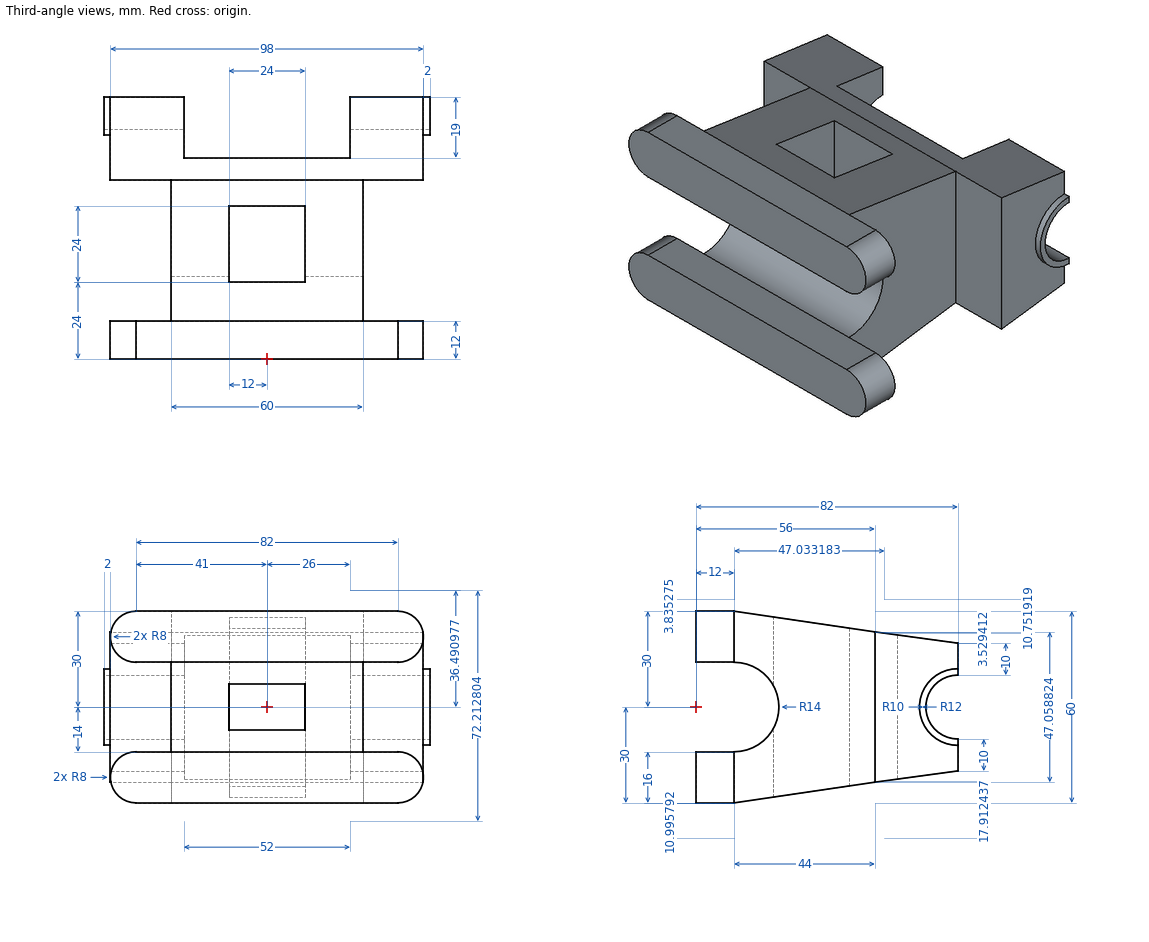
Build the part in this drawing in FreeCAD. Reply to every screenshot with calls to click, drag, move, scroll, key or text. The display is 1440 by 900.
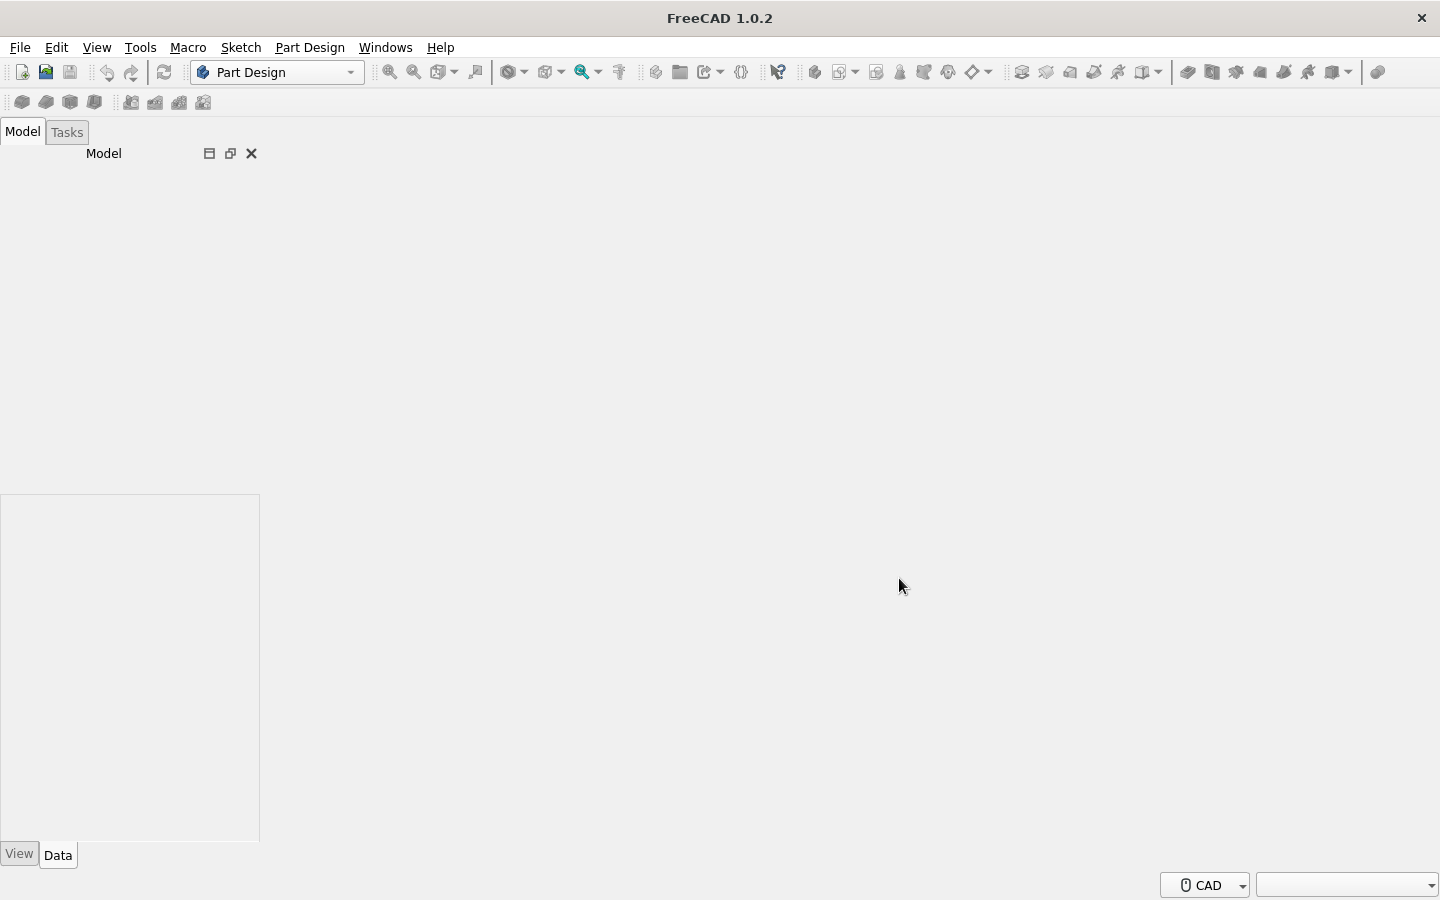
click(22, 72)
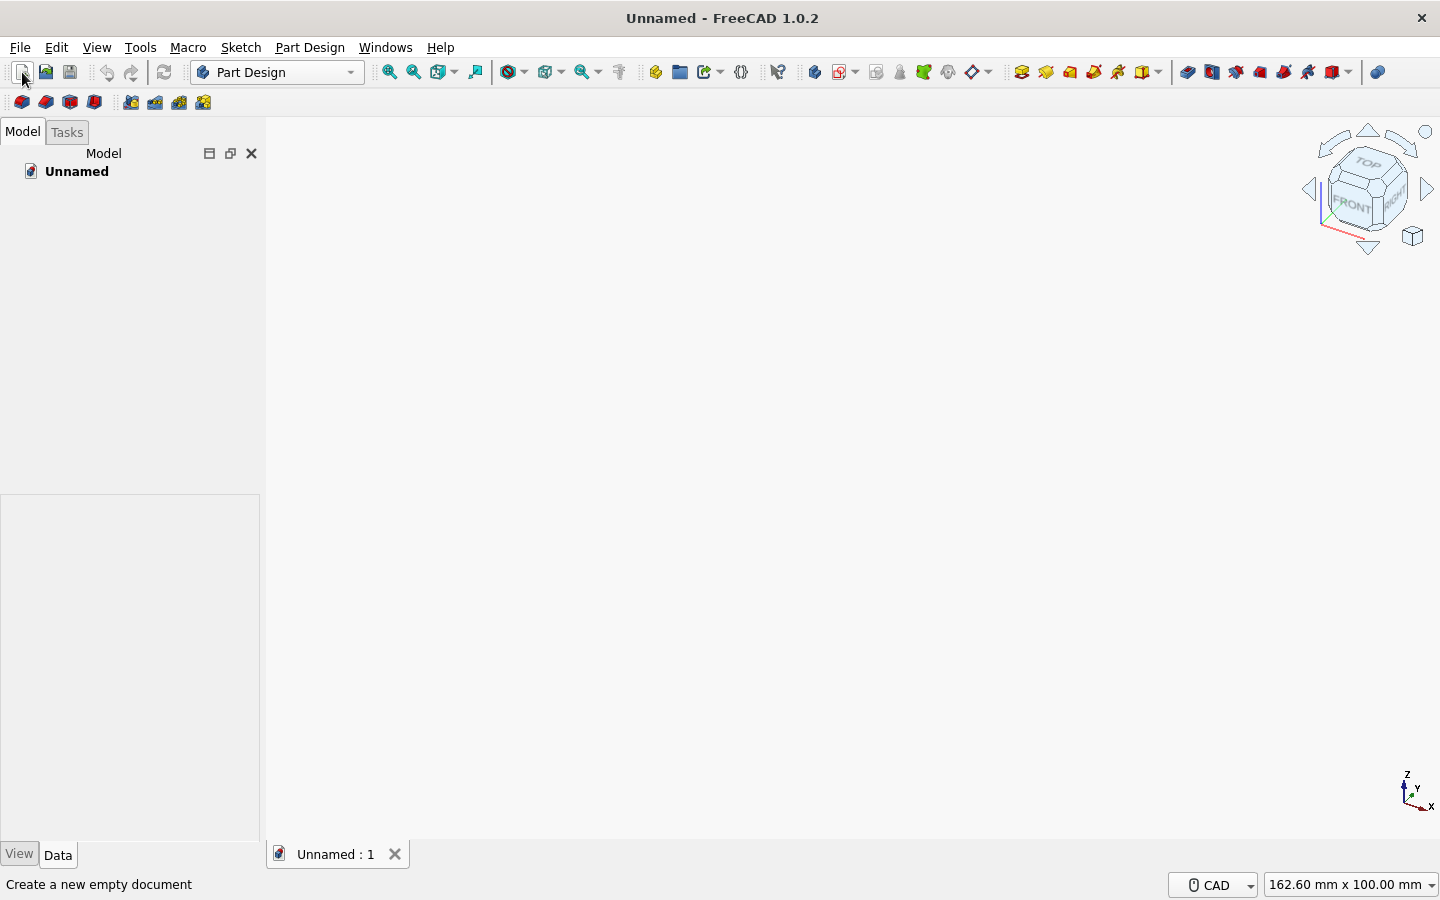
click(840, 72)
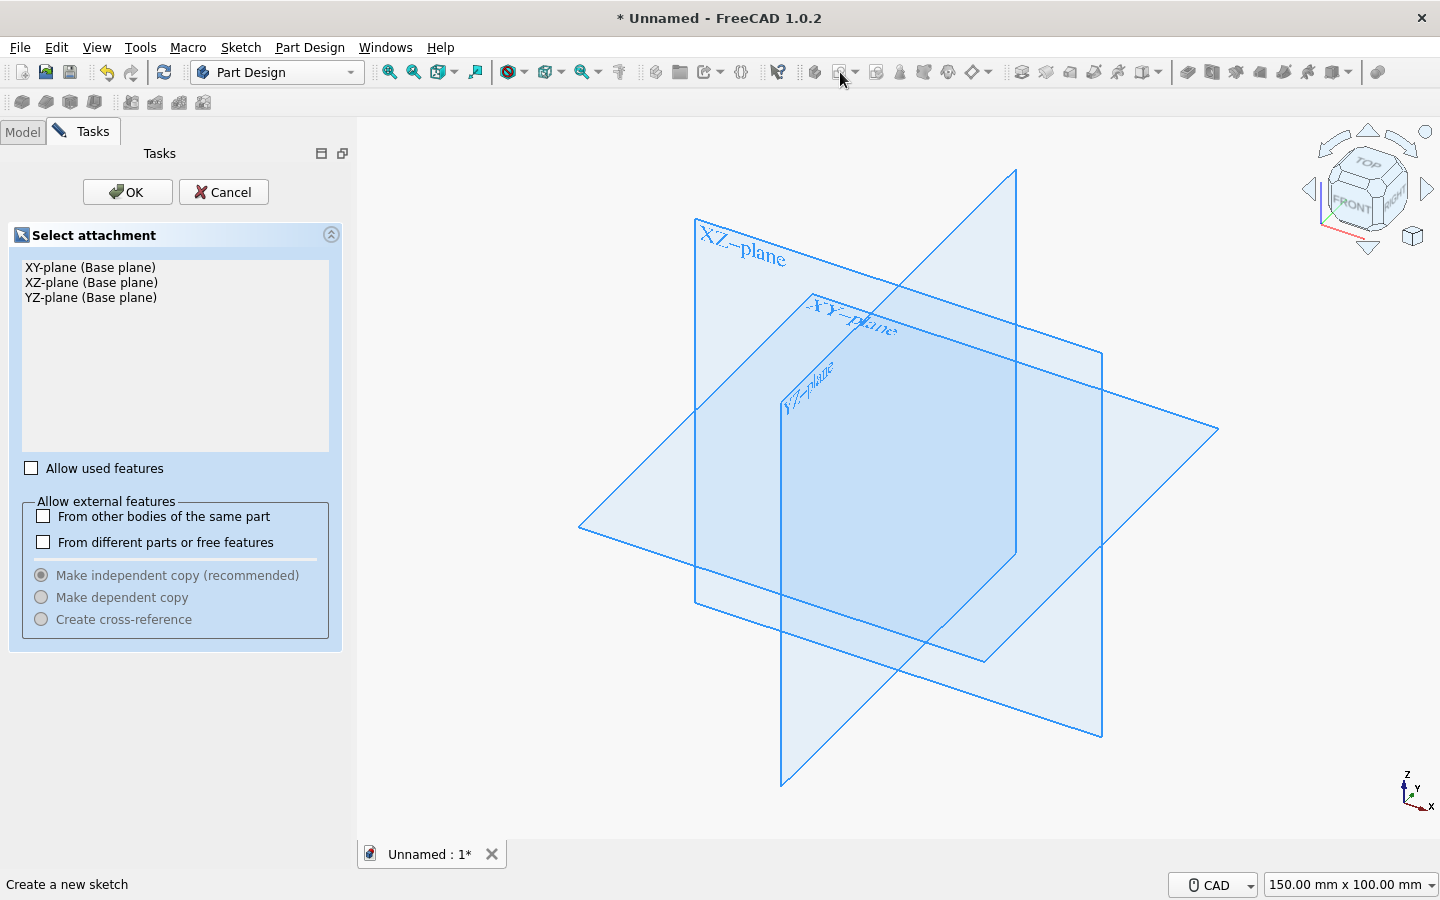
click(82, 282)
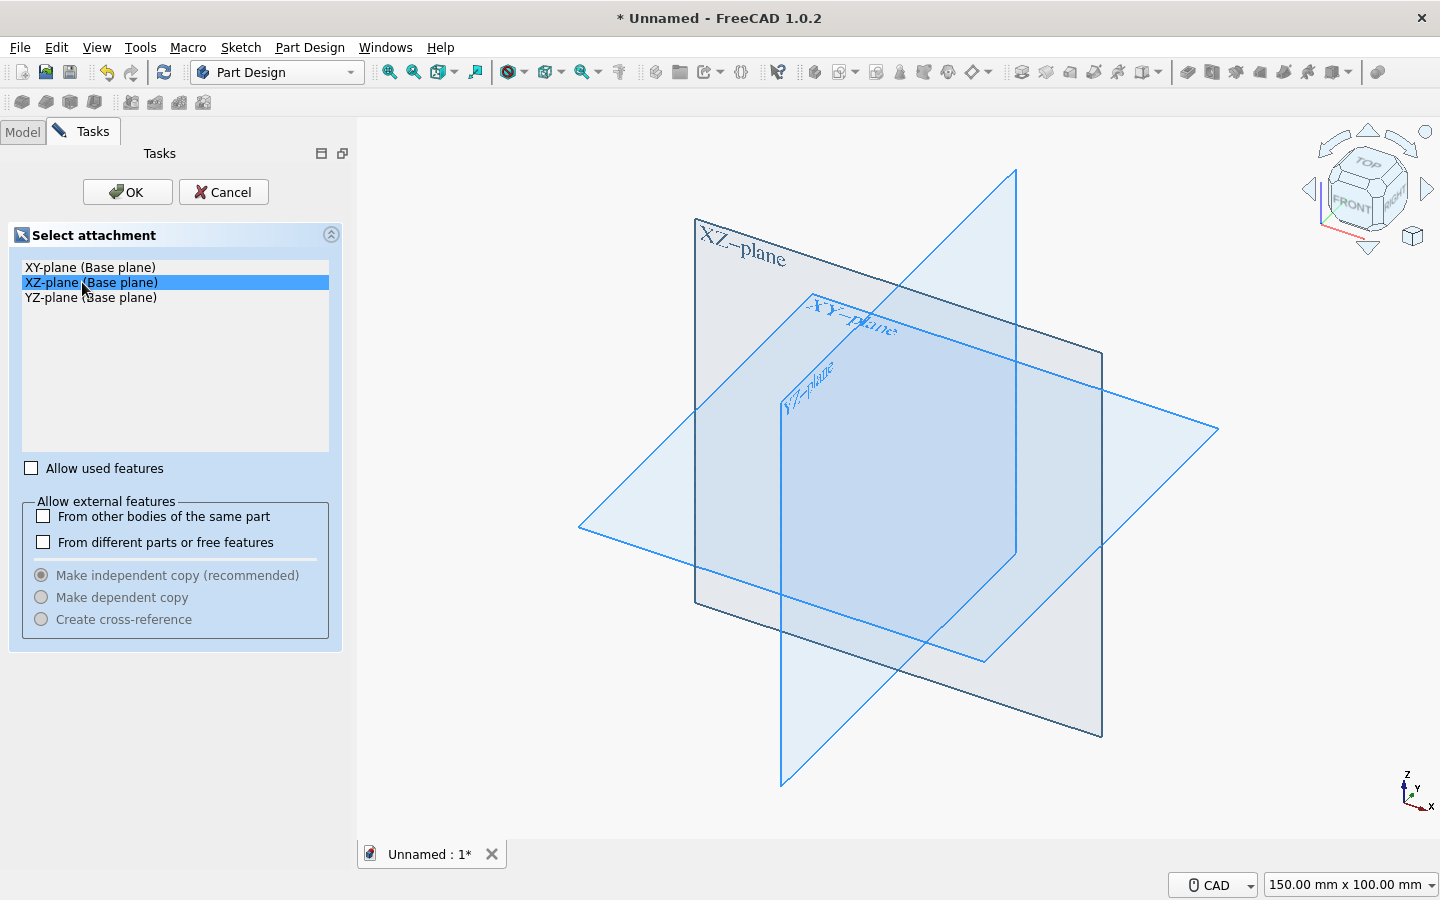
click(128, 192)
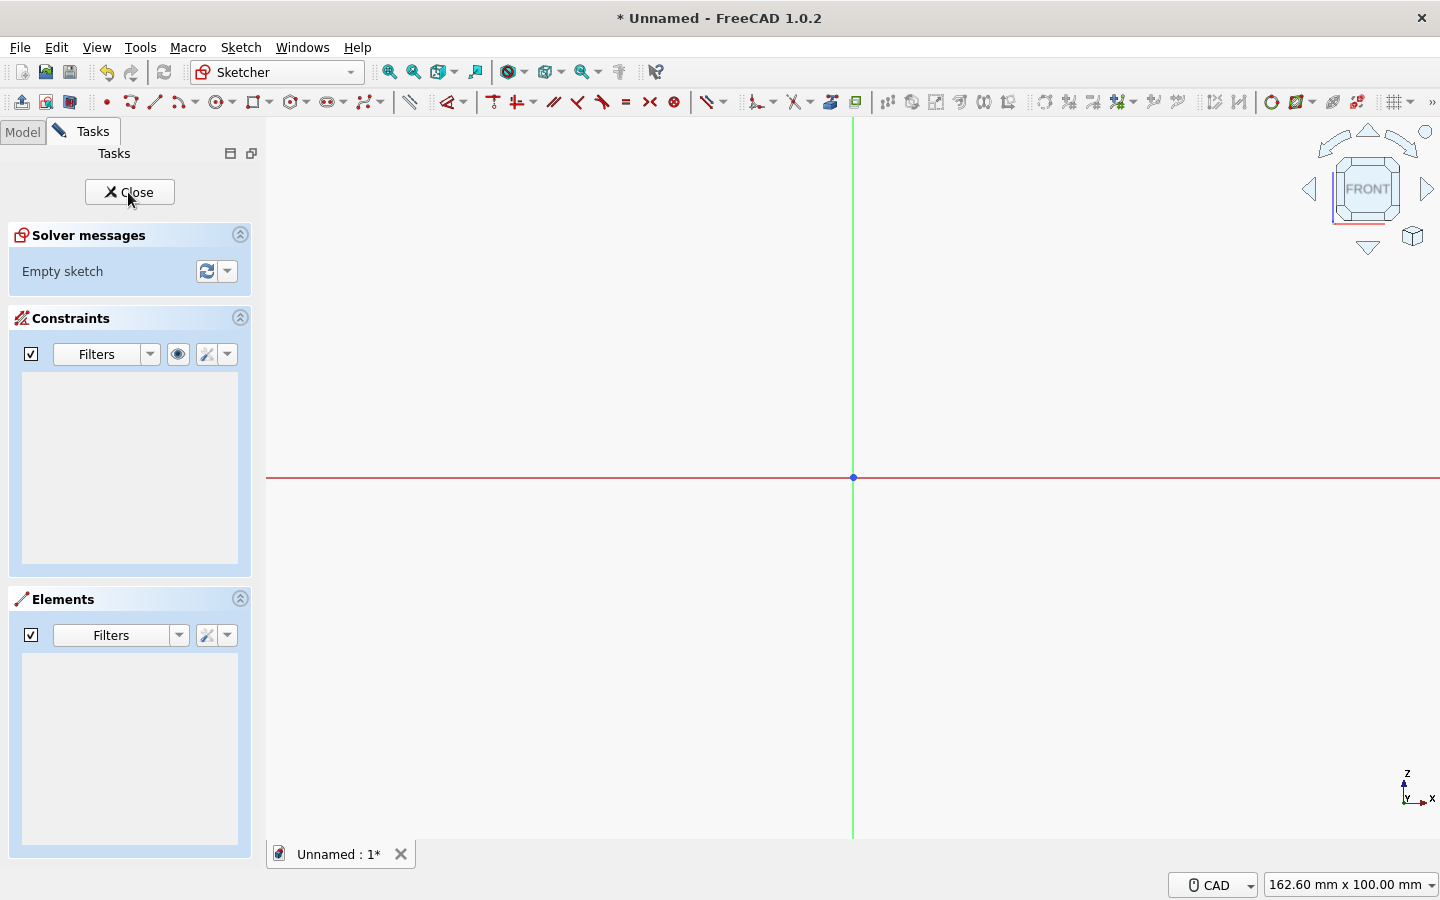
click(328, 102)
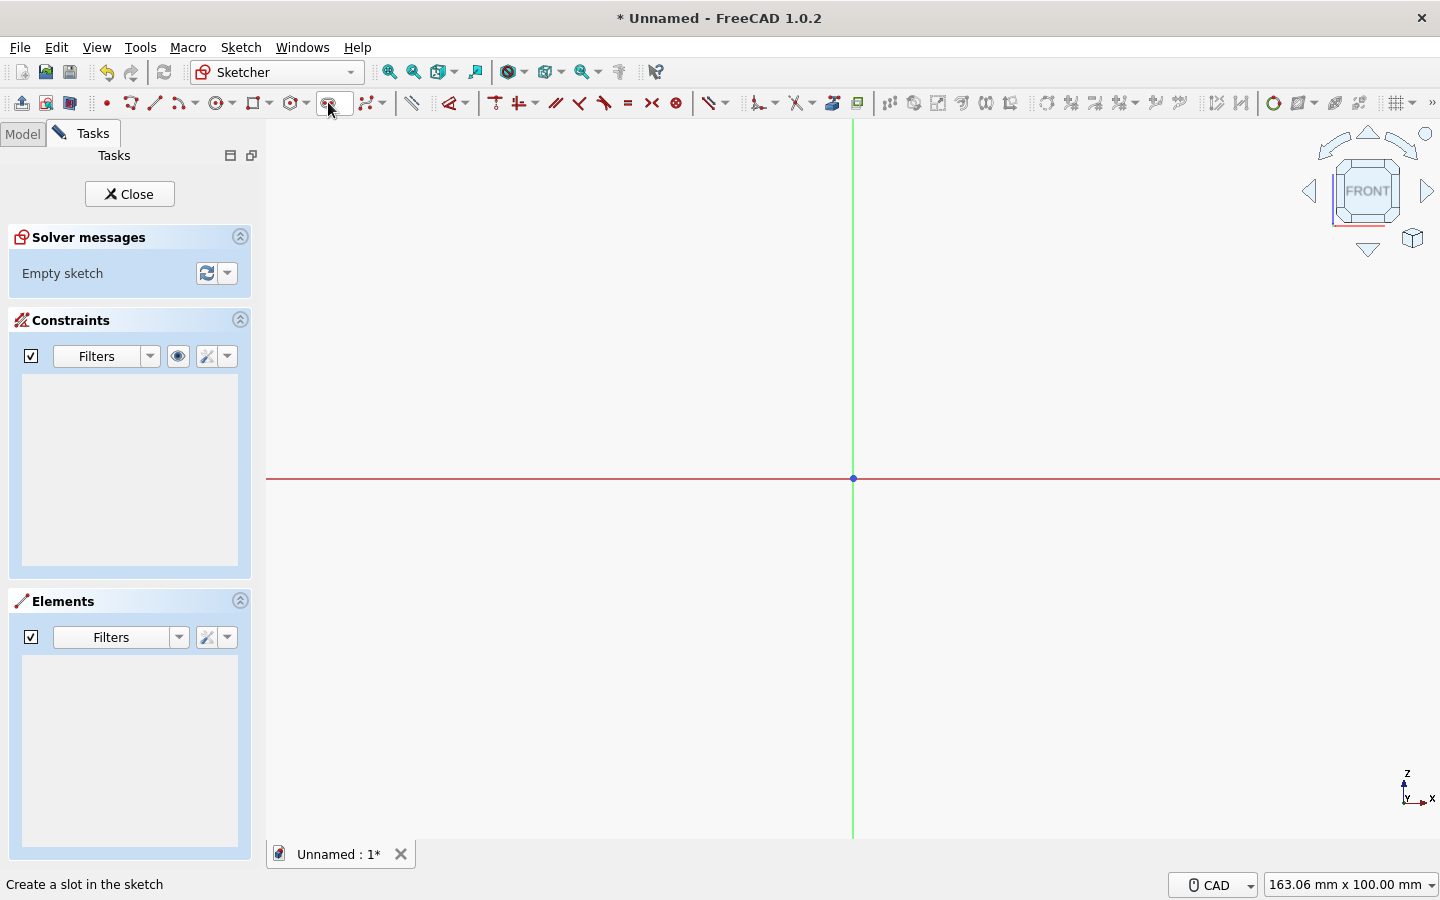
click(558, 321)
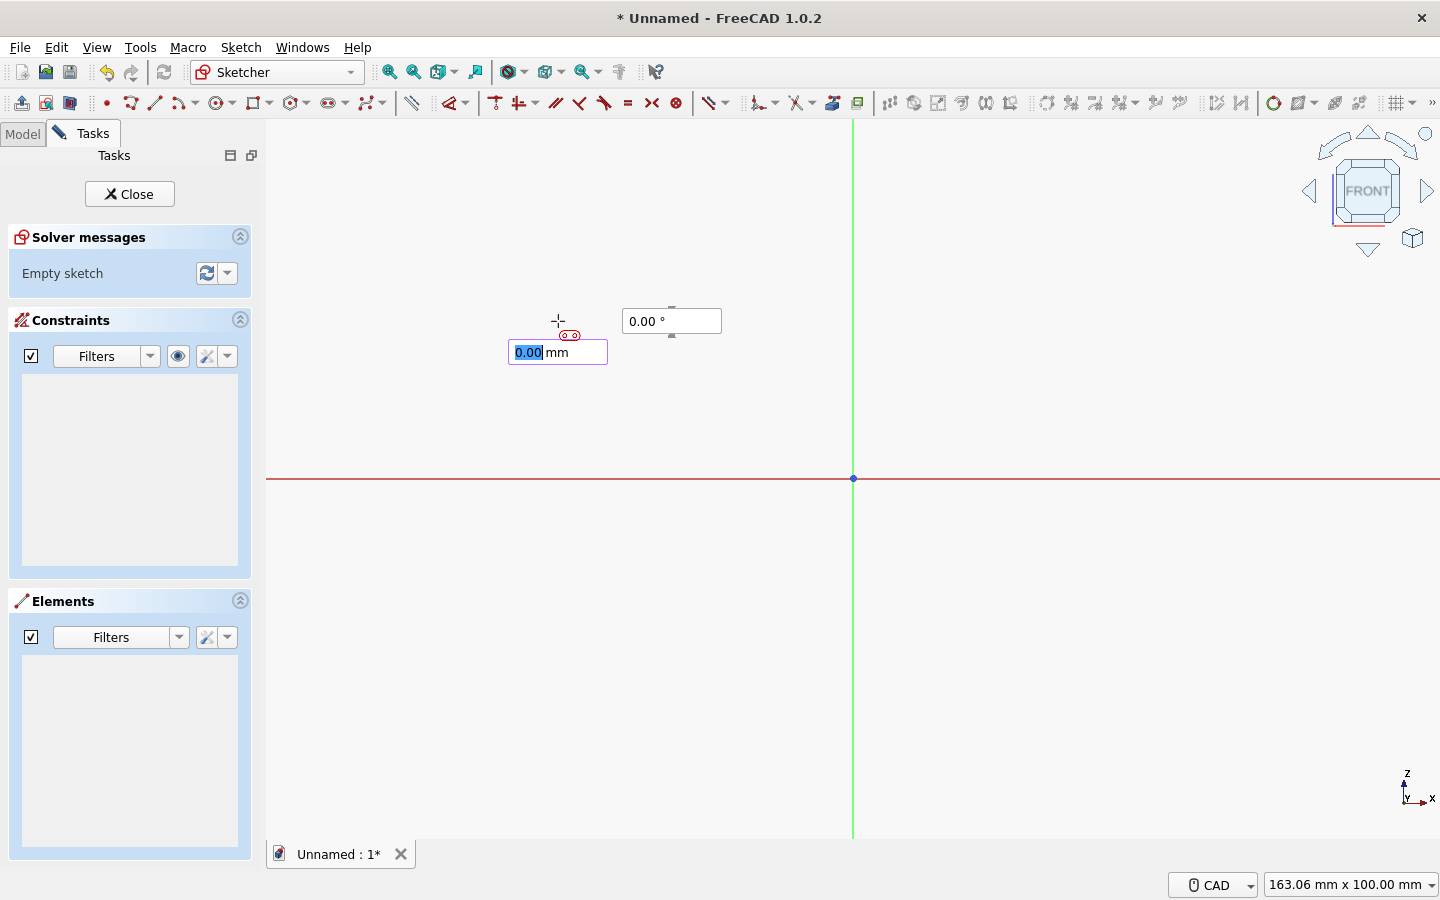
click(1148, 321)